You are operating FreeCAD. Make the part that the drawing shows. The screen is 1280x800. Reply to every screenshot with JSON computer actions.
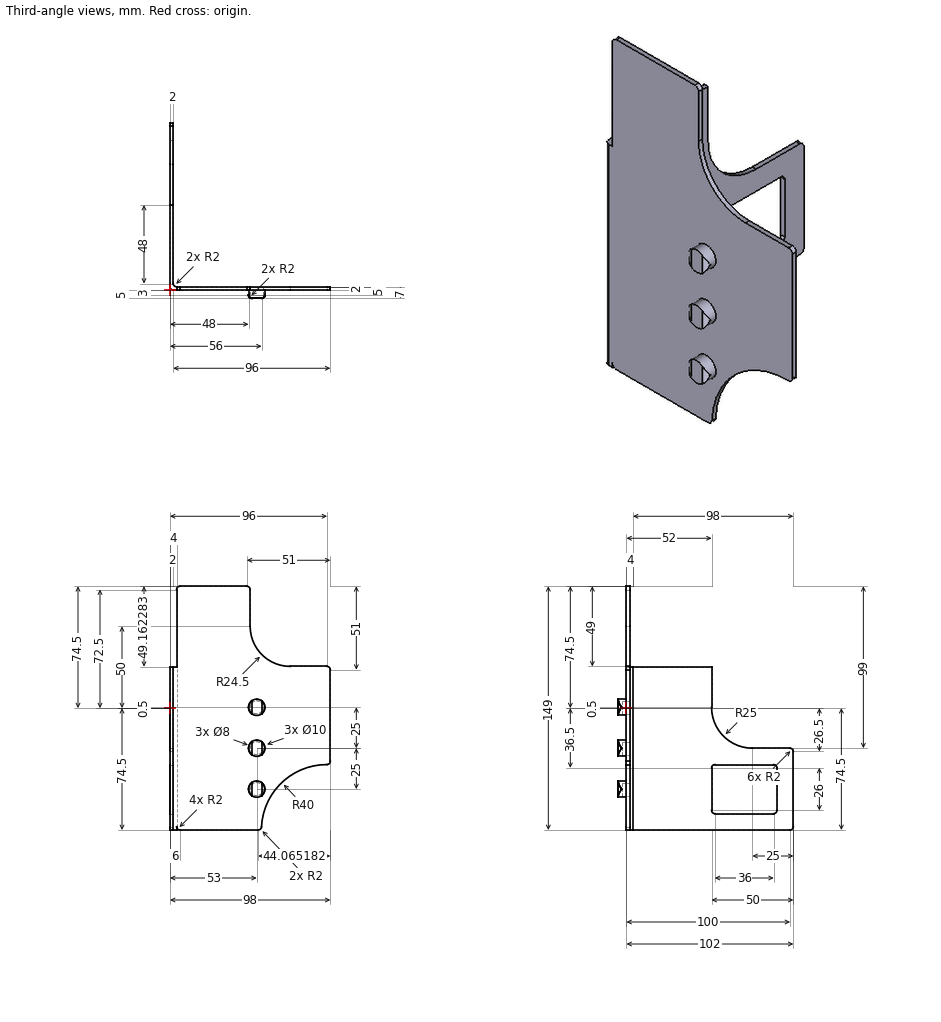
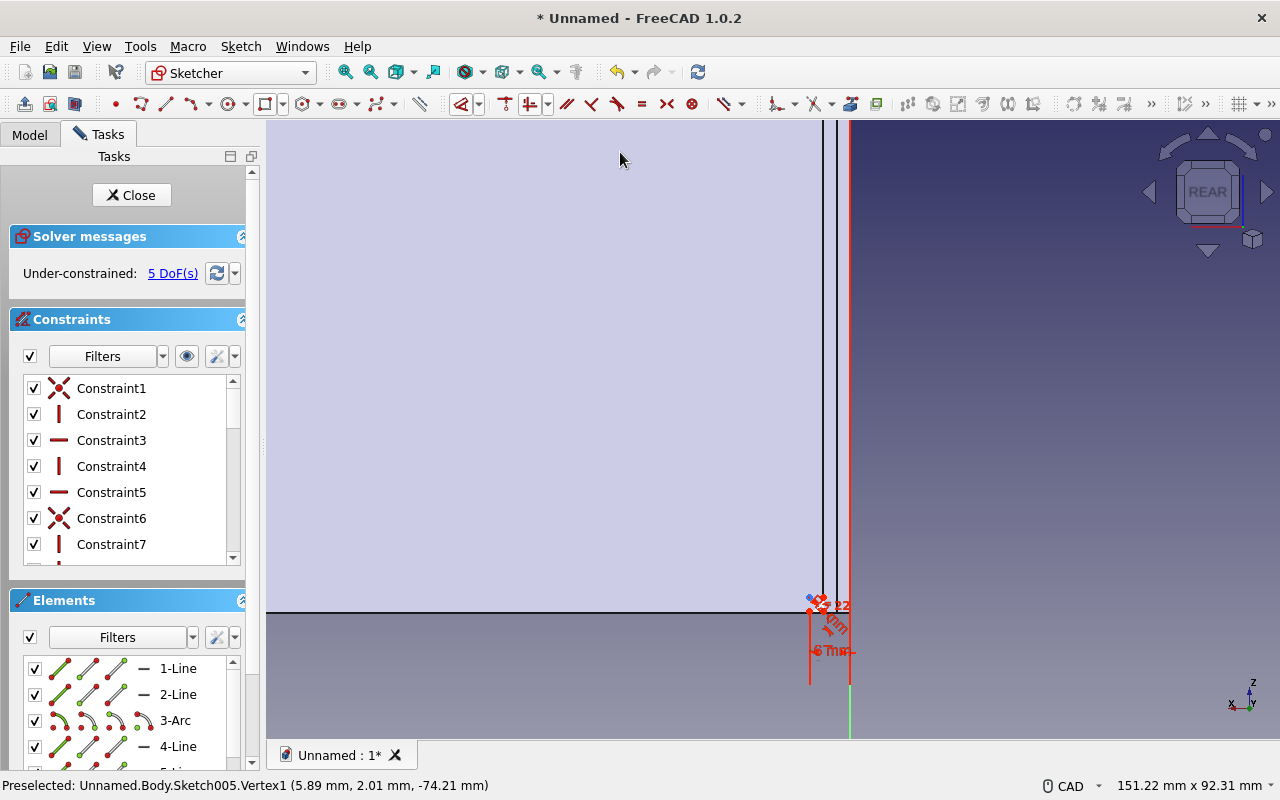
{"action": "scroll", "coordinate": [811, 613], "scroll_direction": "down", "scroll_amount": 5}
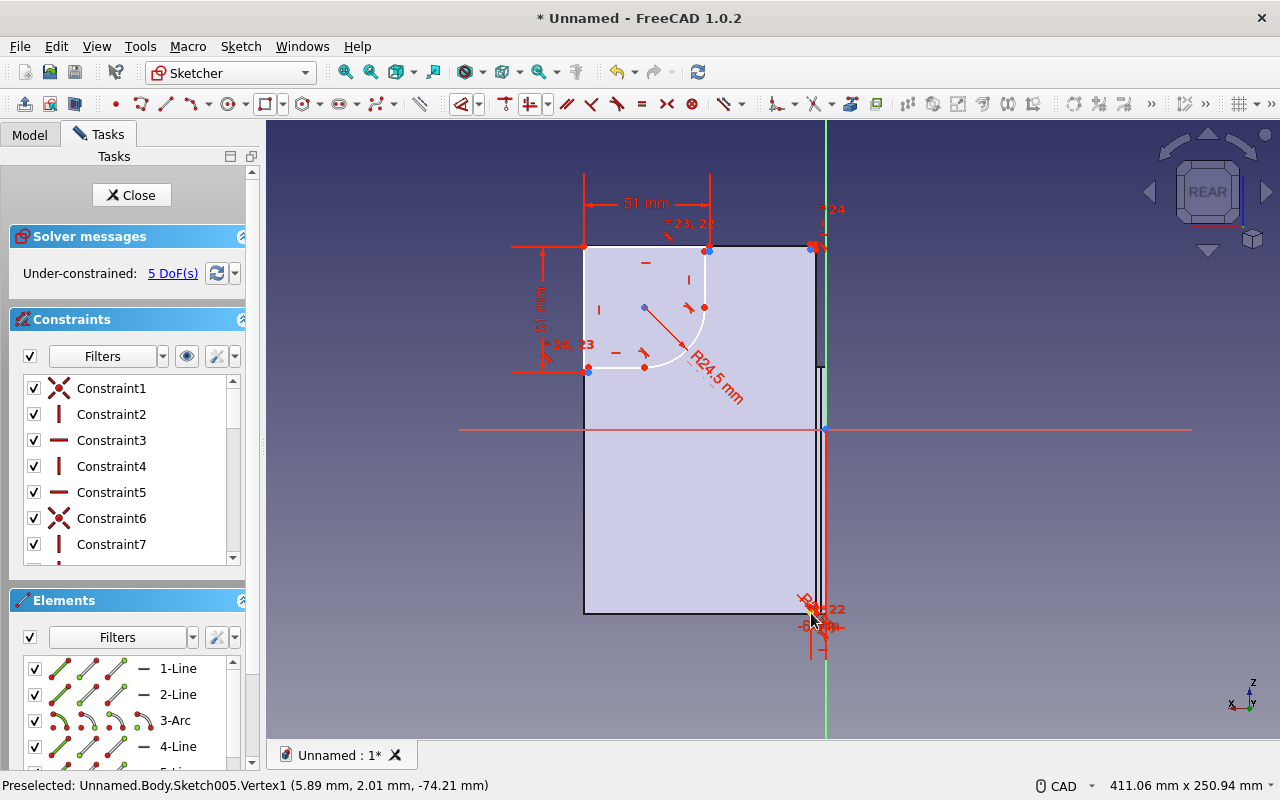
{"action": "scroll", "coordinate": [816, 249], "scroll_direction": "up", "scroll_amount": 7}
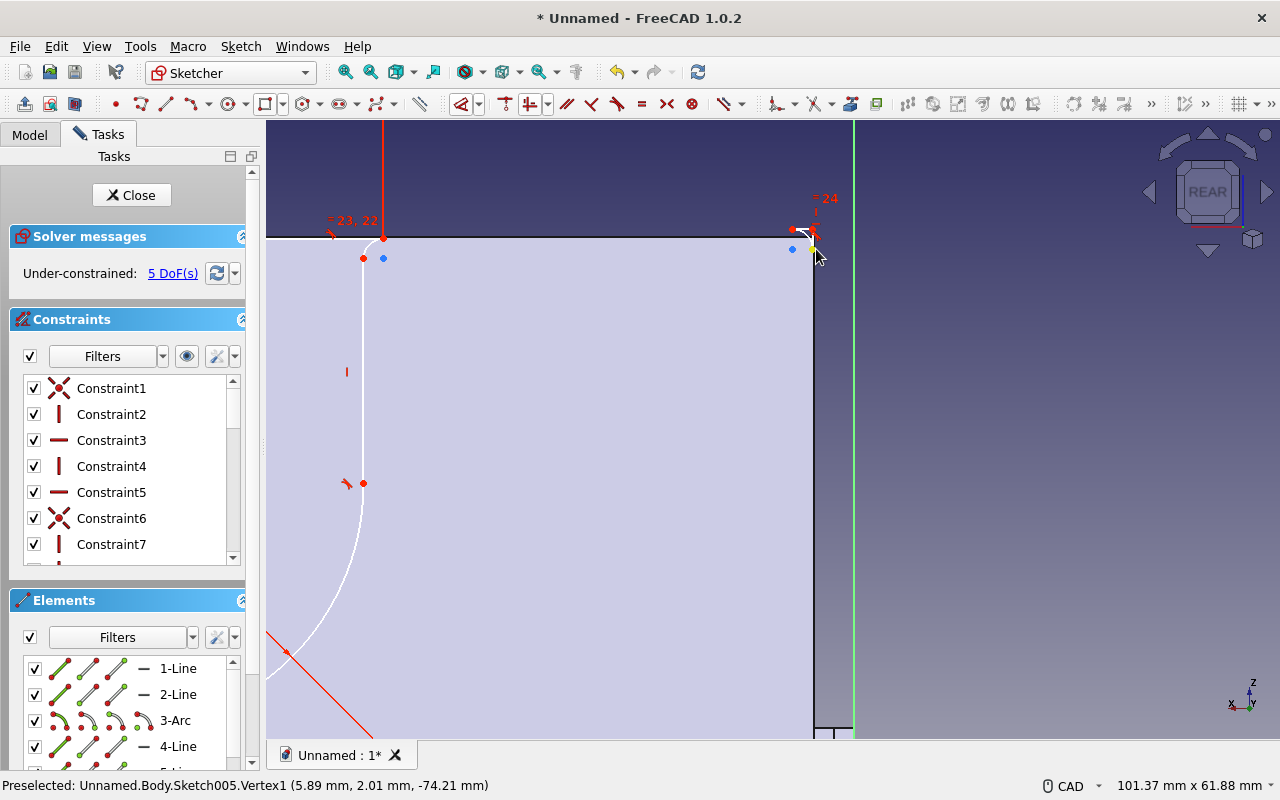
{"action": "left_click", "coordinate": [813, 249]}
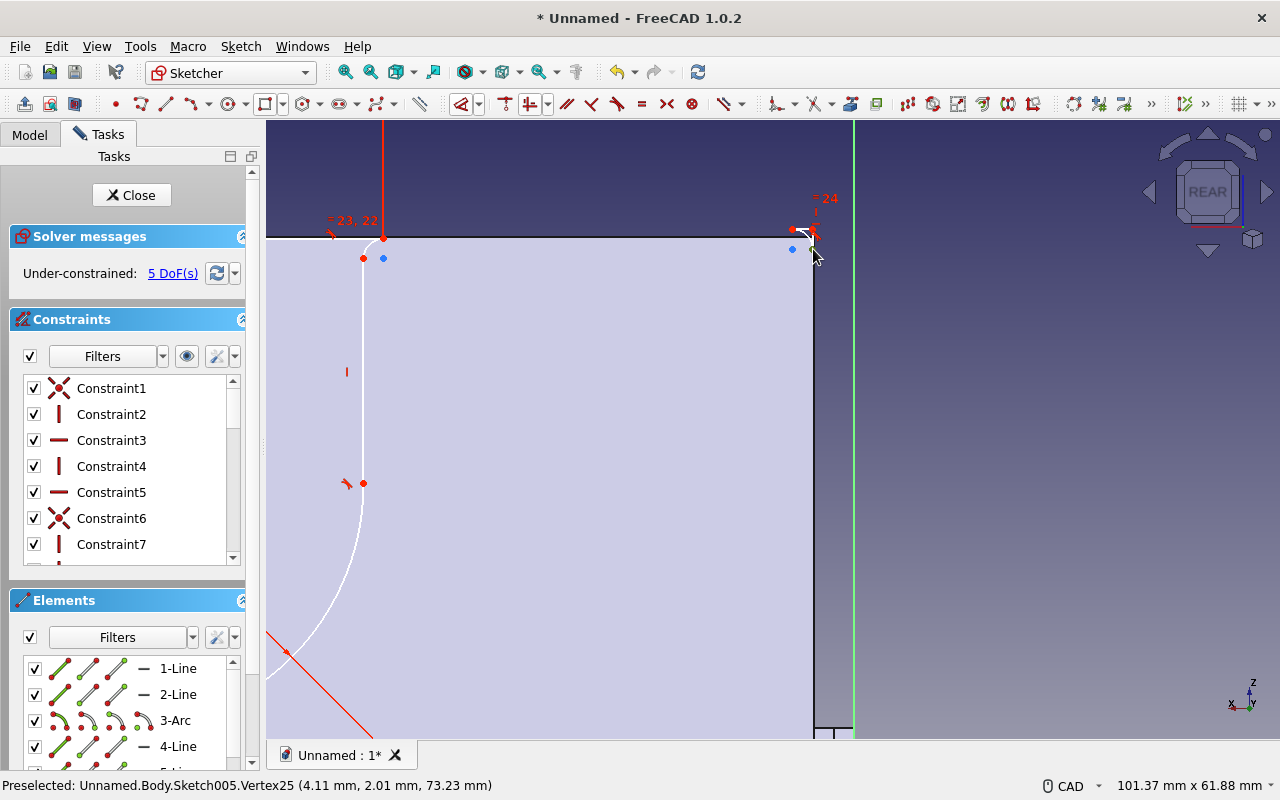
{"action": "left_click", "coordinate": [478, 104]}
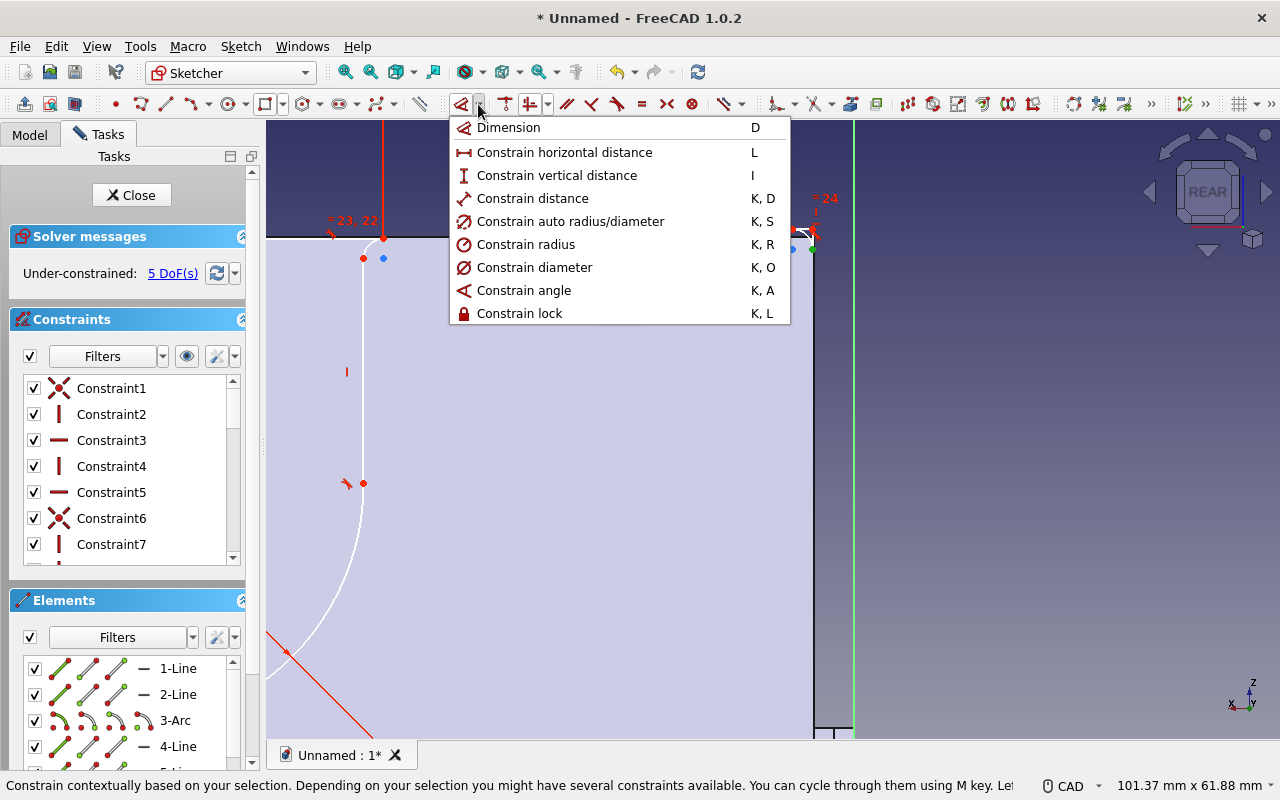
{"action": "left_click", "coordinate": [620, 152]}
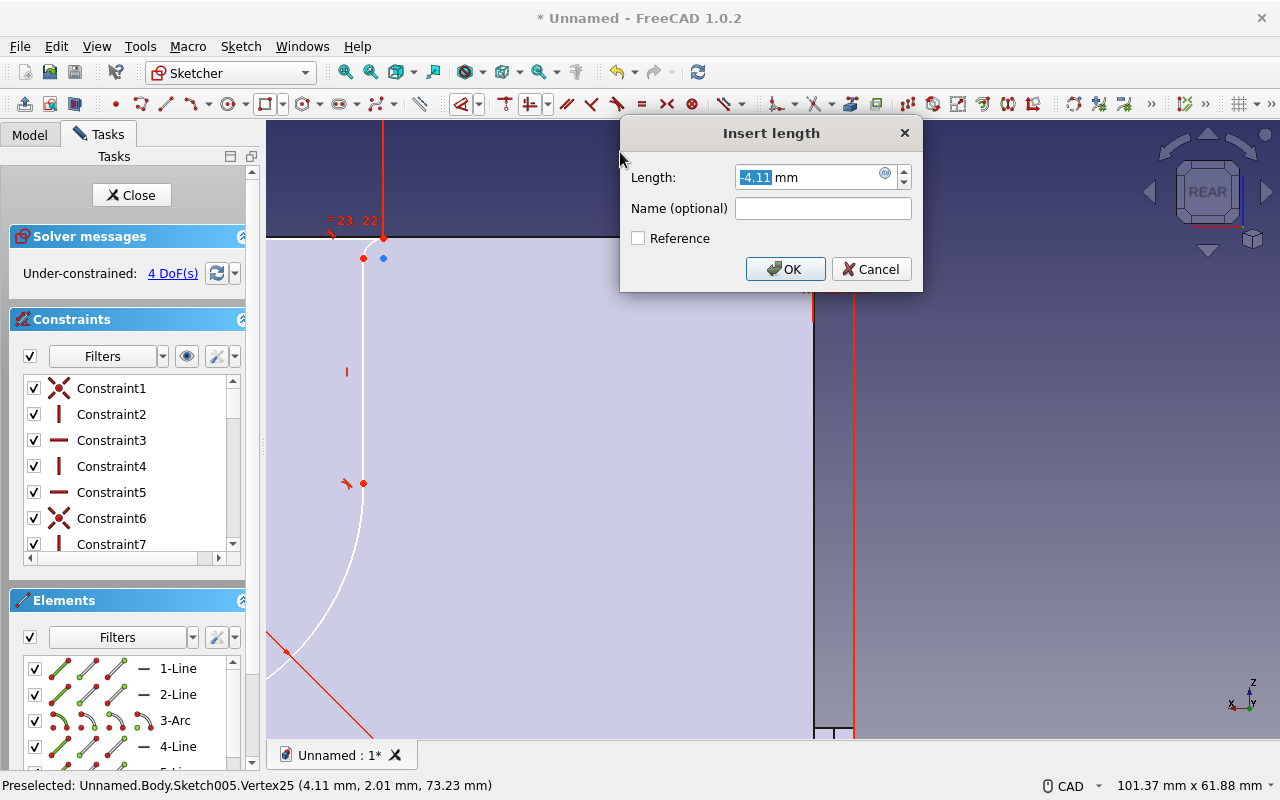
{"action": "type", "text": "-4"}
{"action": "key", "text": "Return"}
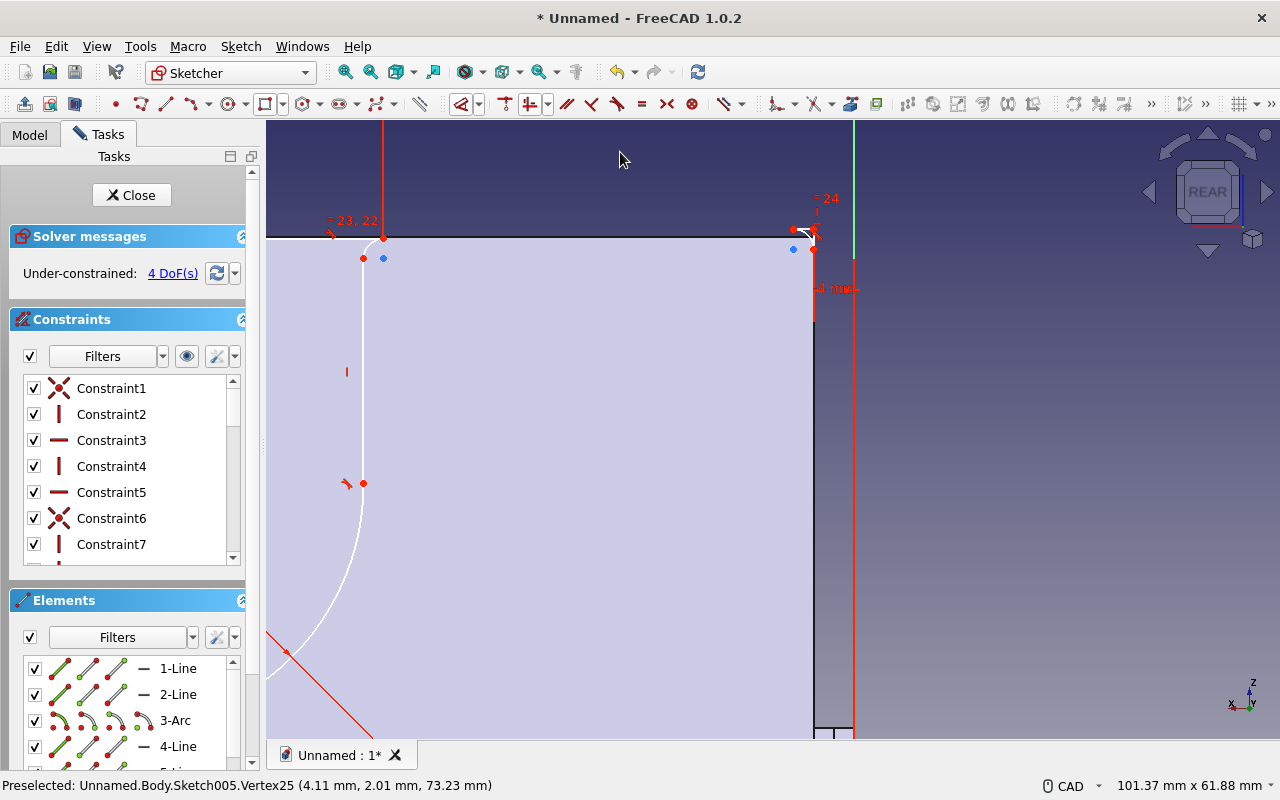
{"action": "scroll", "coordinate": [816, 249], "scroll_direction": "down", "scroll_amount": 7}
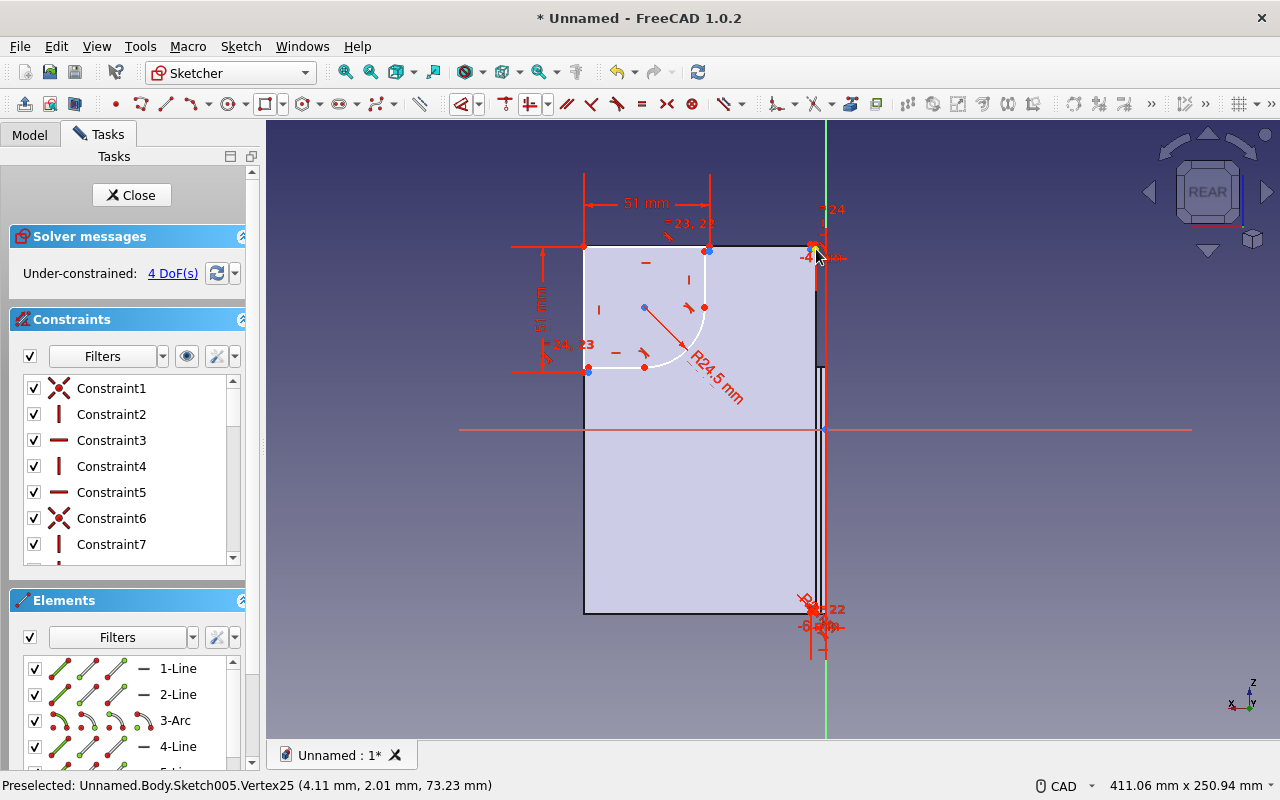
{"action": "scroll", "coordinate": [589, 368], "scroll_direction": "up", "scroll_amount": 5}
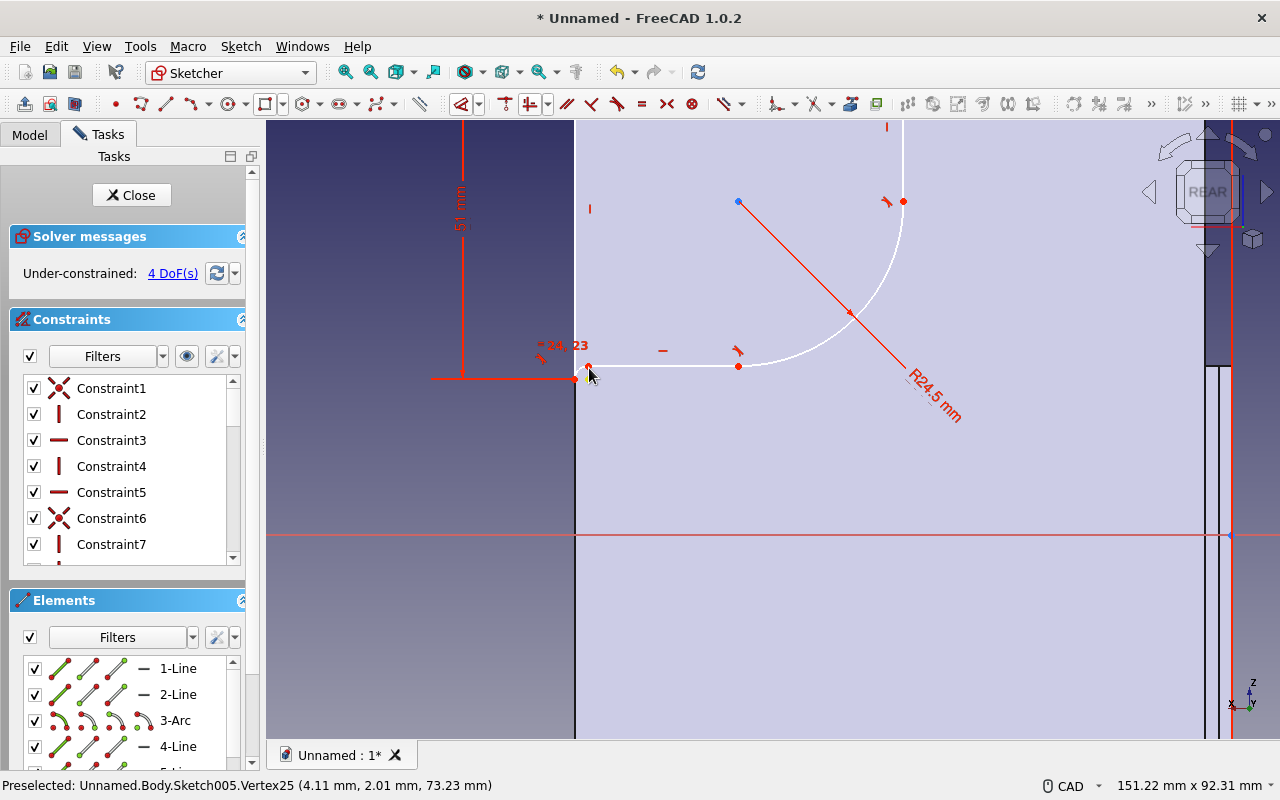
{"action": "left_click", "coordinate": [588, 366]}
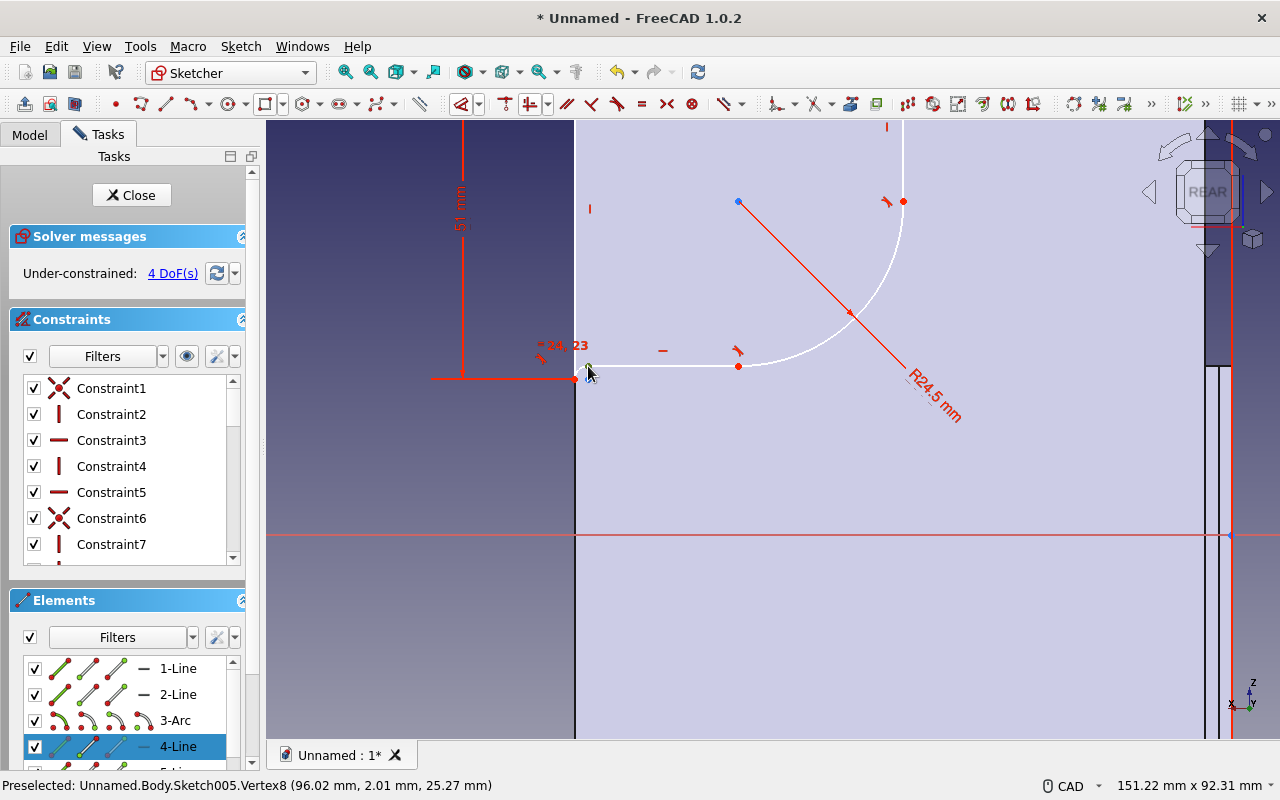
{"action": "key", "text": "l"}